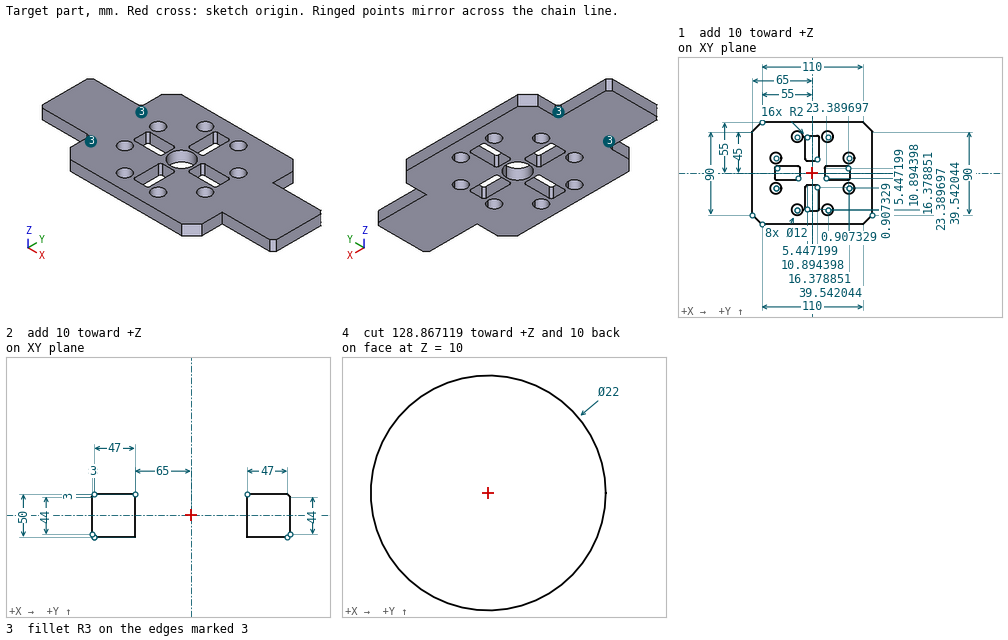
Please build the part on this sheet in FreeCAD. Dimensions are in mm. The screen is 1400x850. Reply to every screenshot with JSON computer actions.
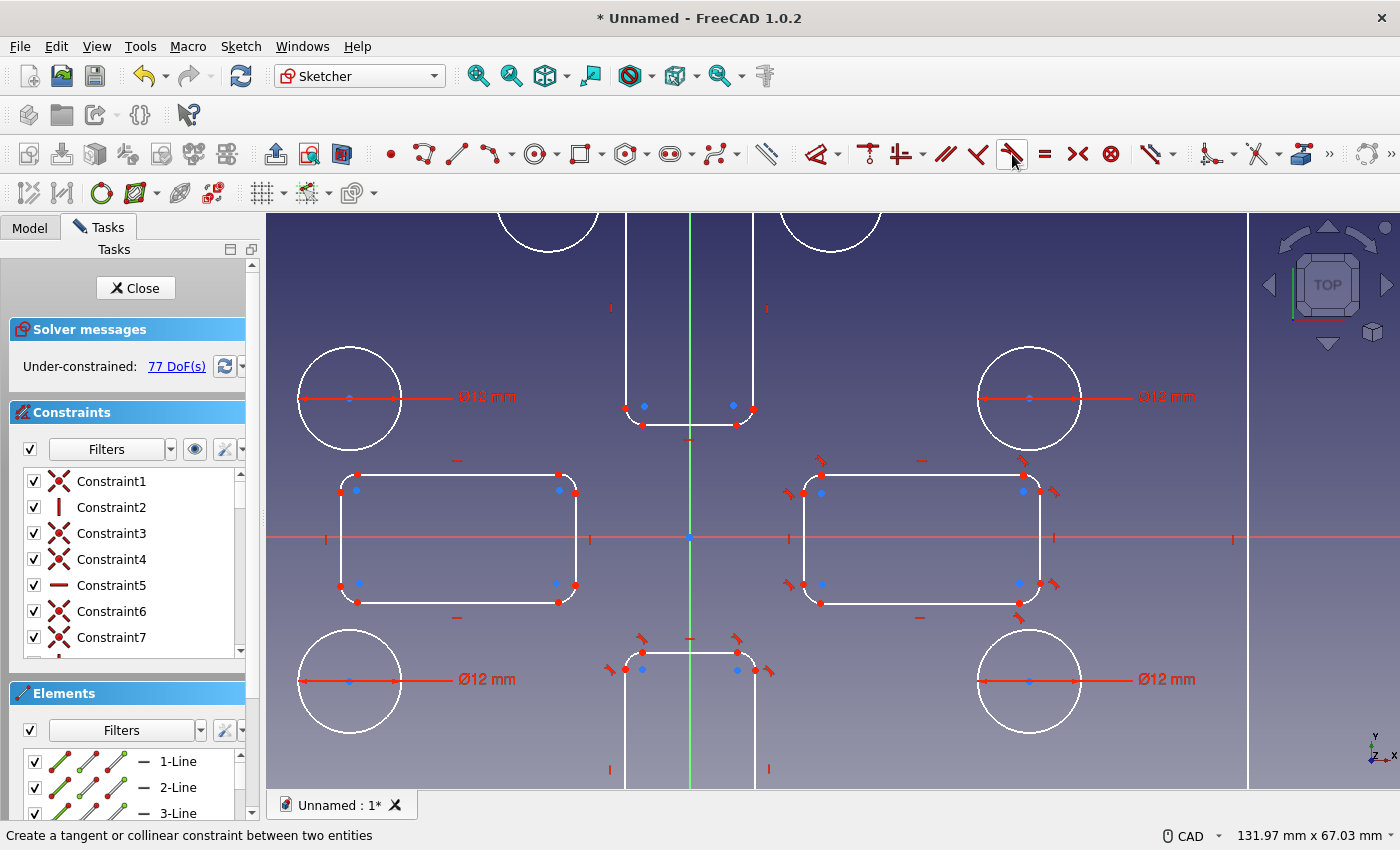
{"action": "left_click", "coordinate": [960, 604]}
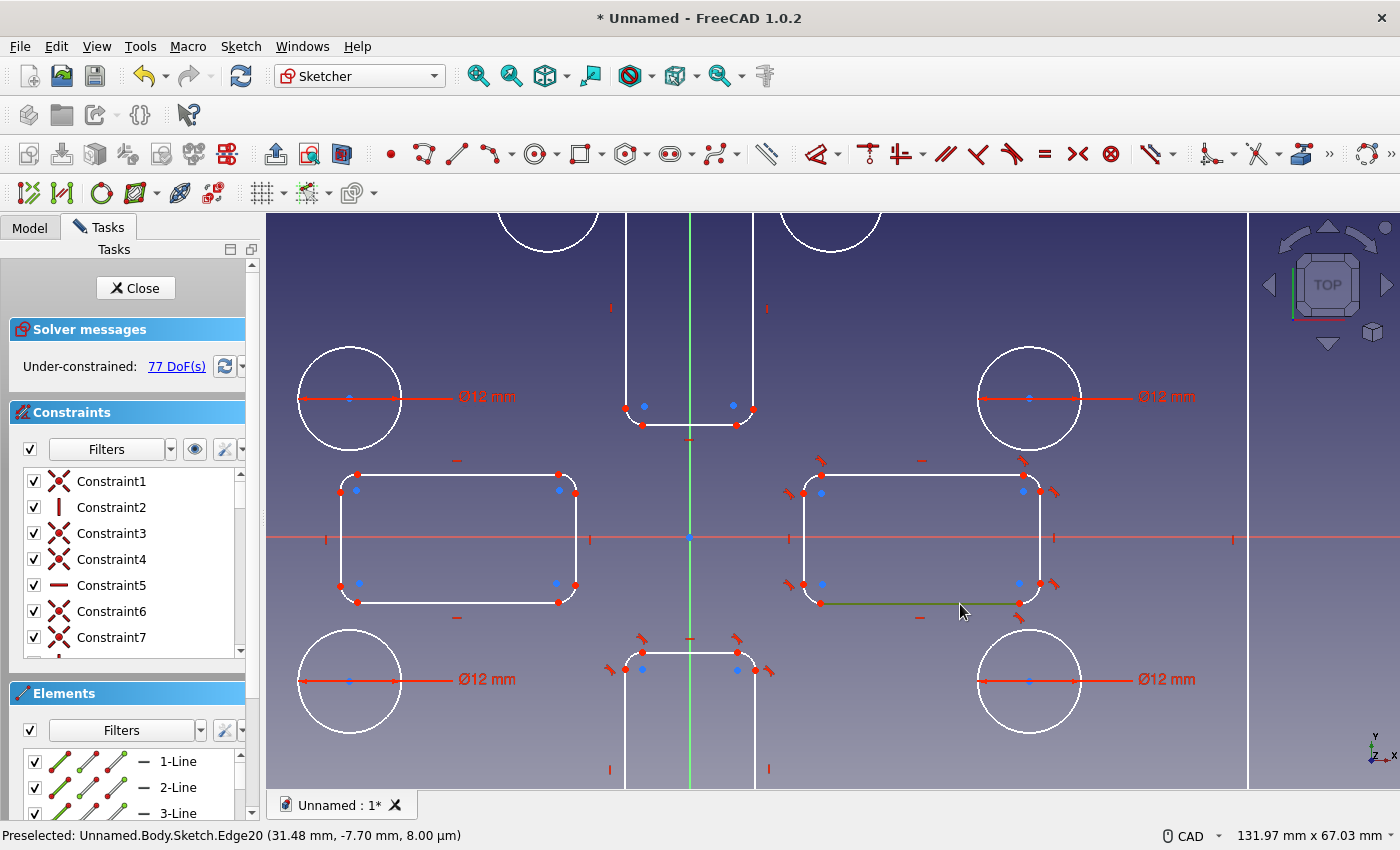
{"action": "left_click", "coordinate": [809, 597]}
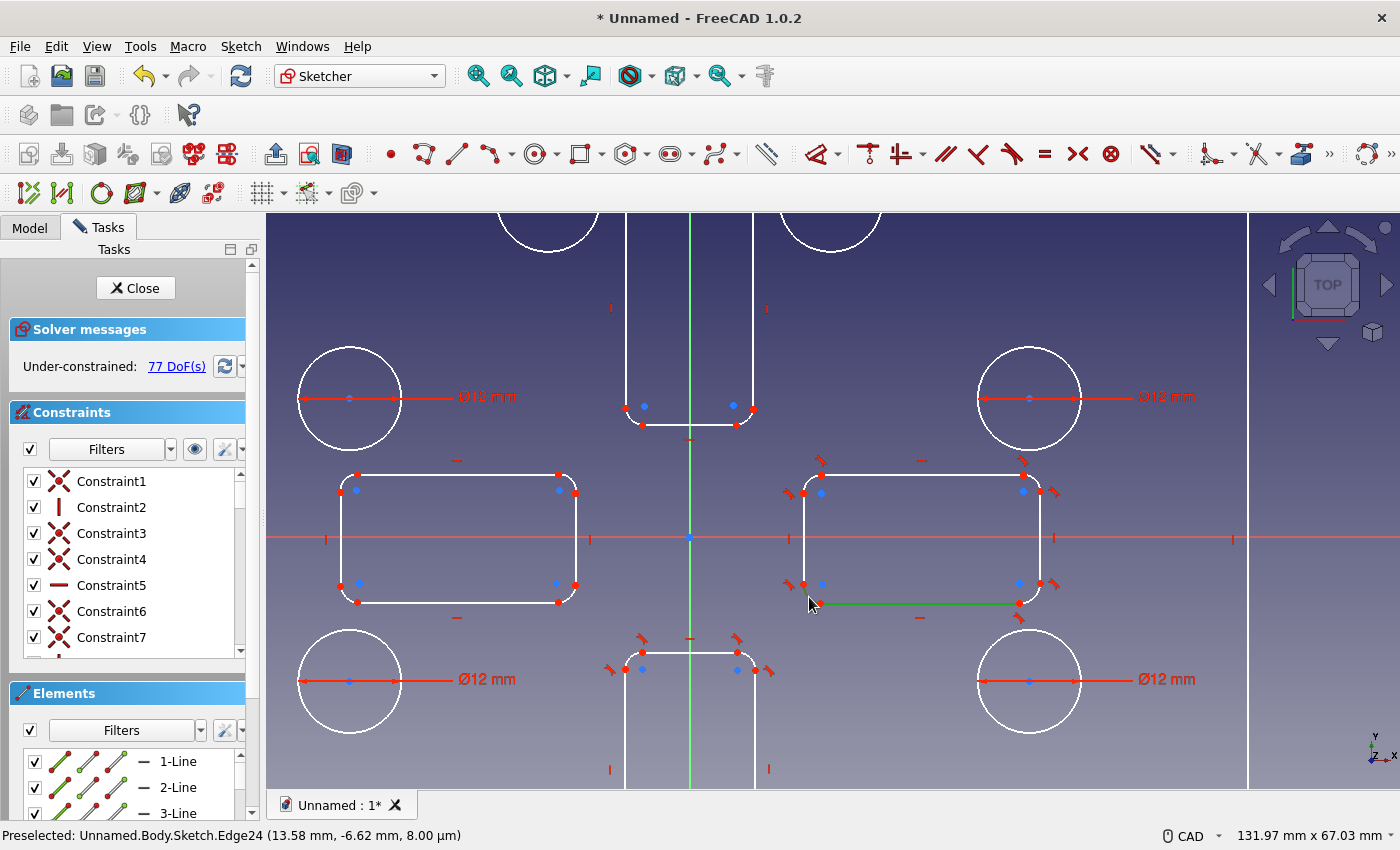
{"action": "left_click", "coordinate": [1012, 154]}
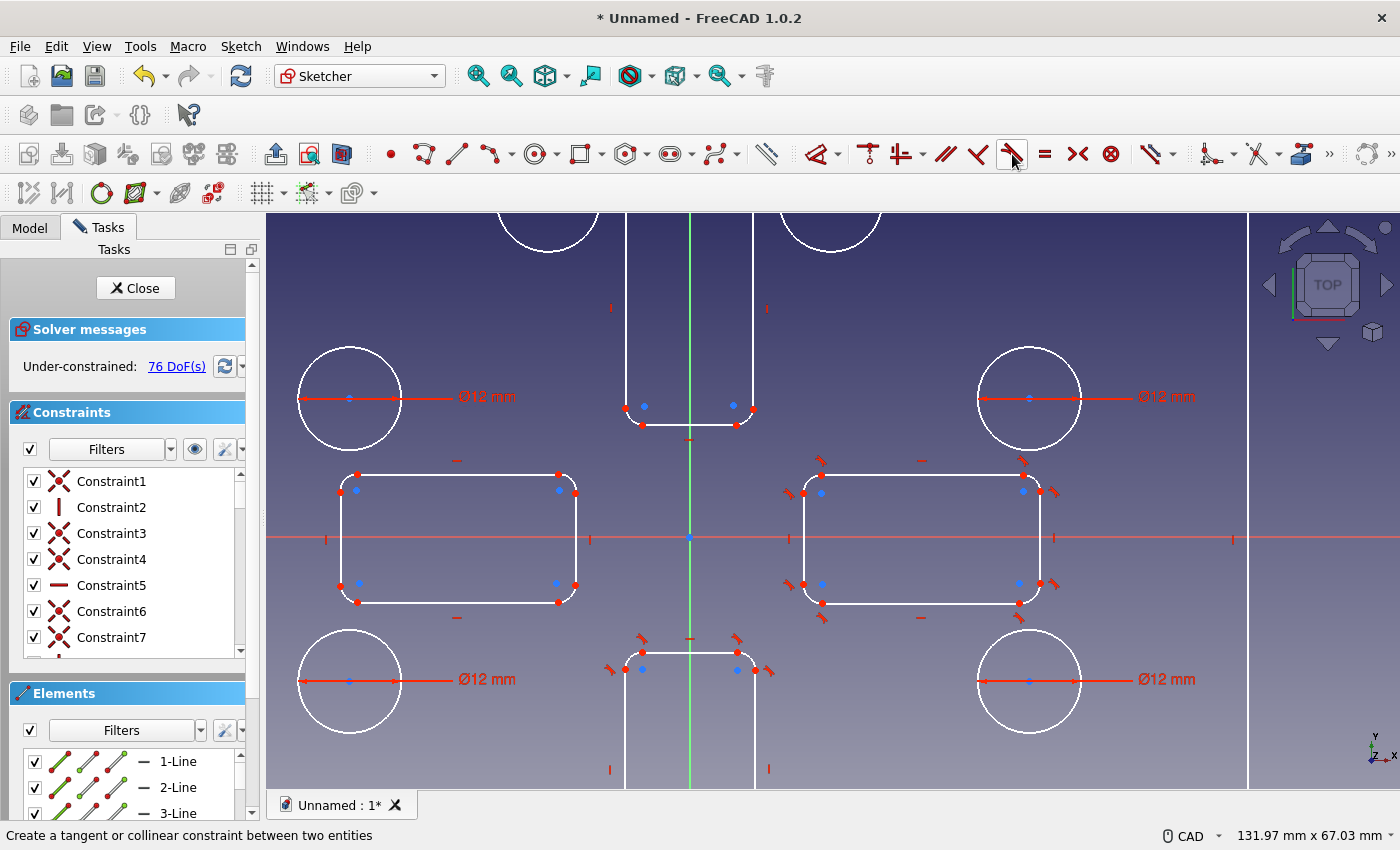
{"action": "left_click", "coordinate": [576, 521]}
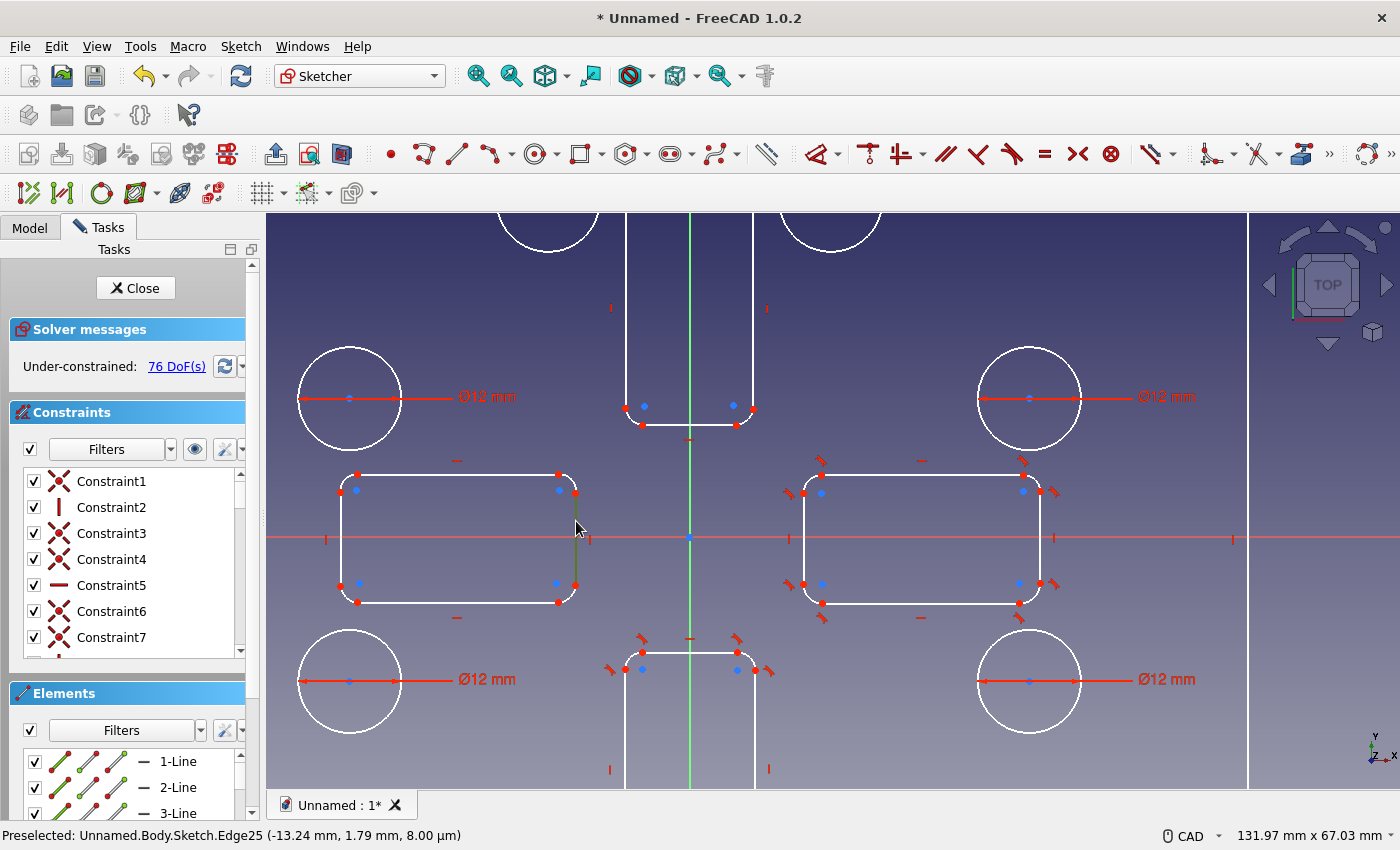
{"action": "left_click", "coordinate": [570, 597]}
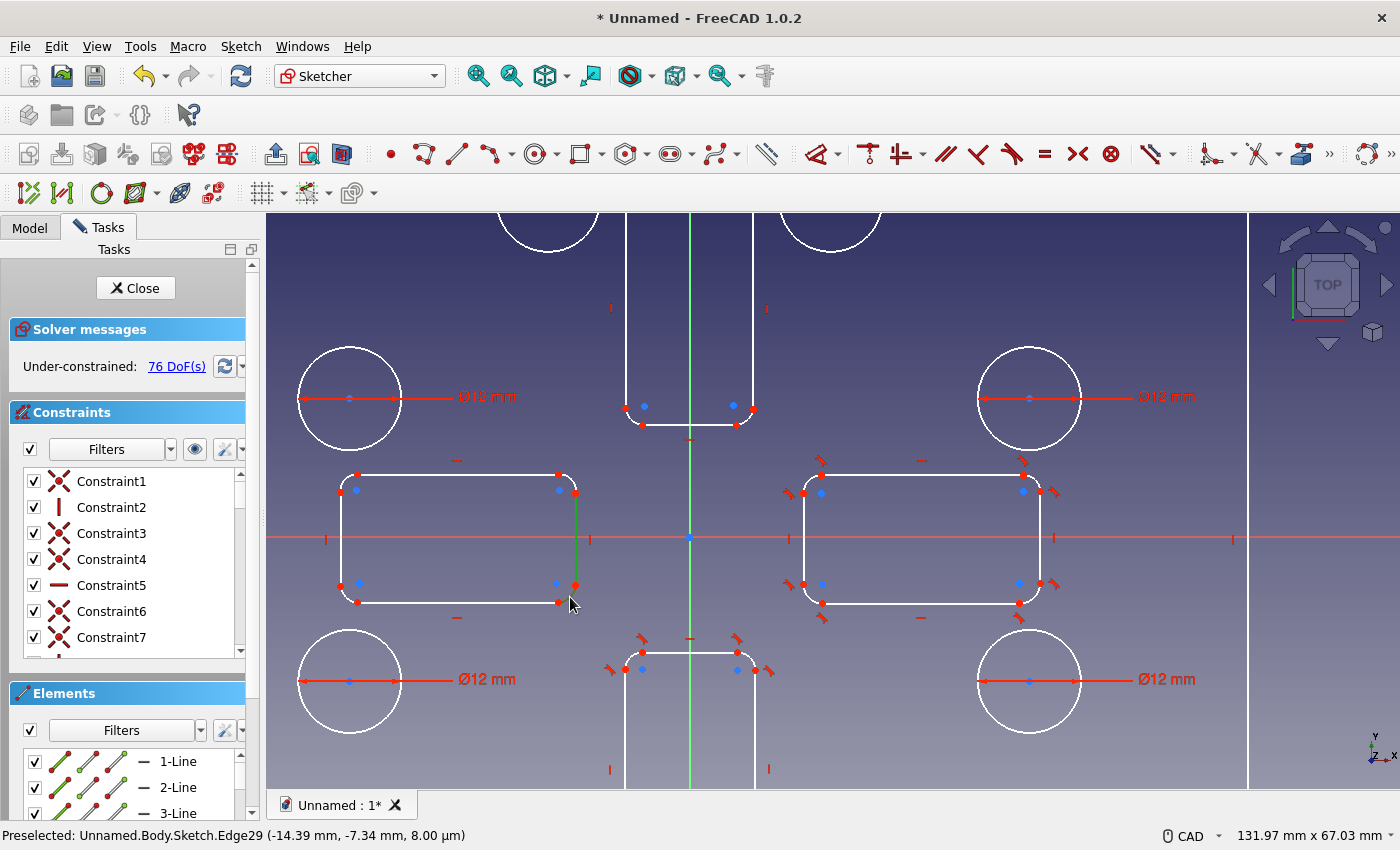
{"action": "left_click", "coordinate": [1012, 154]}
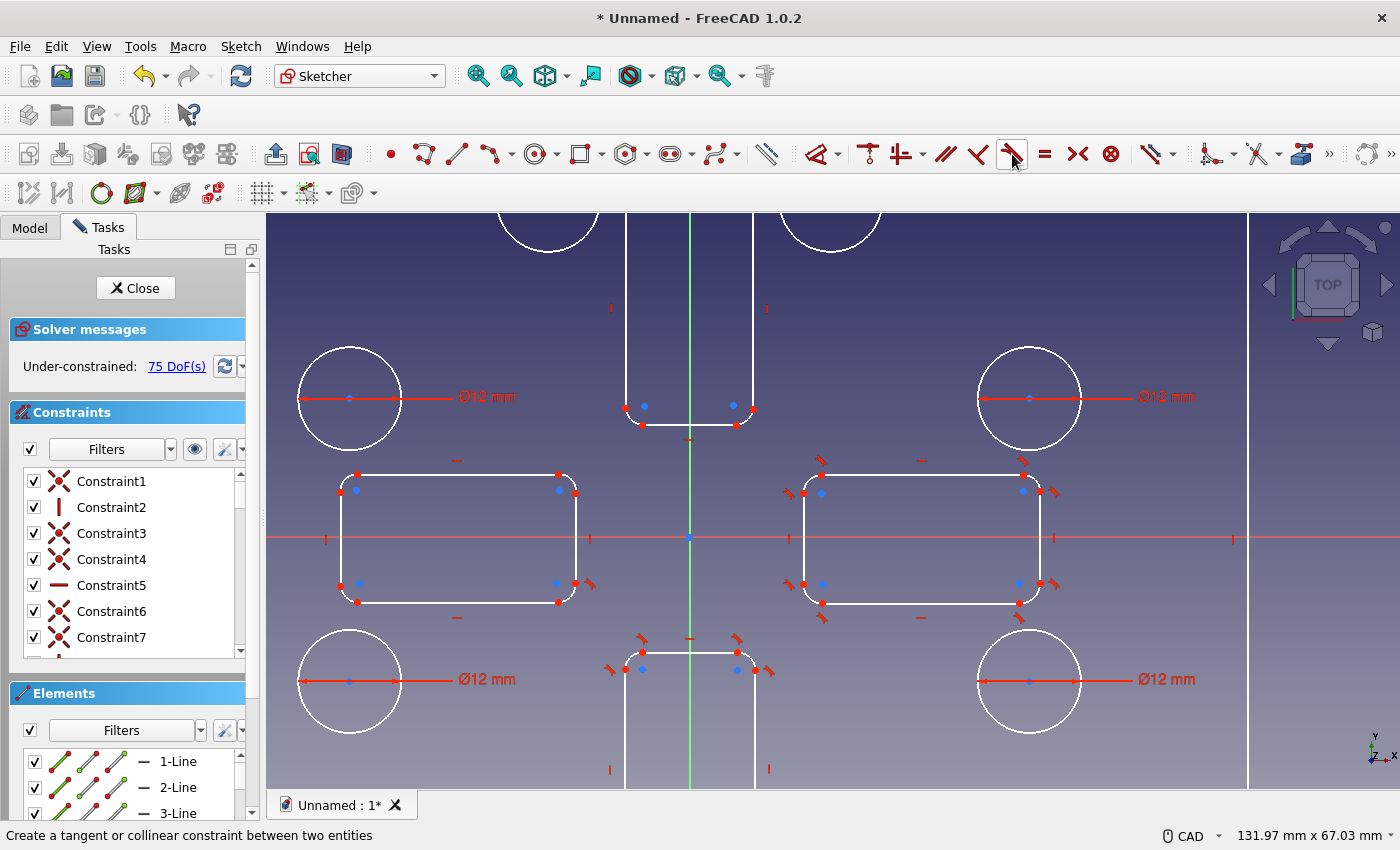
{"action": "left_click", "coordinate": [576, 520]}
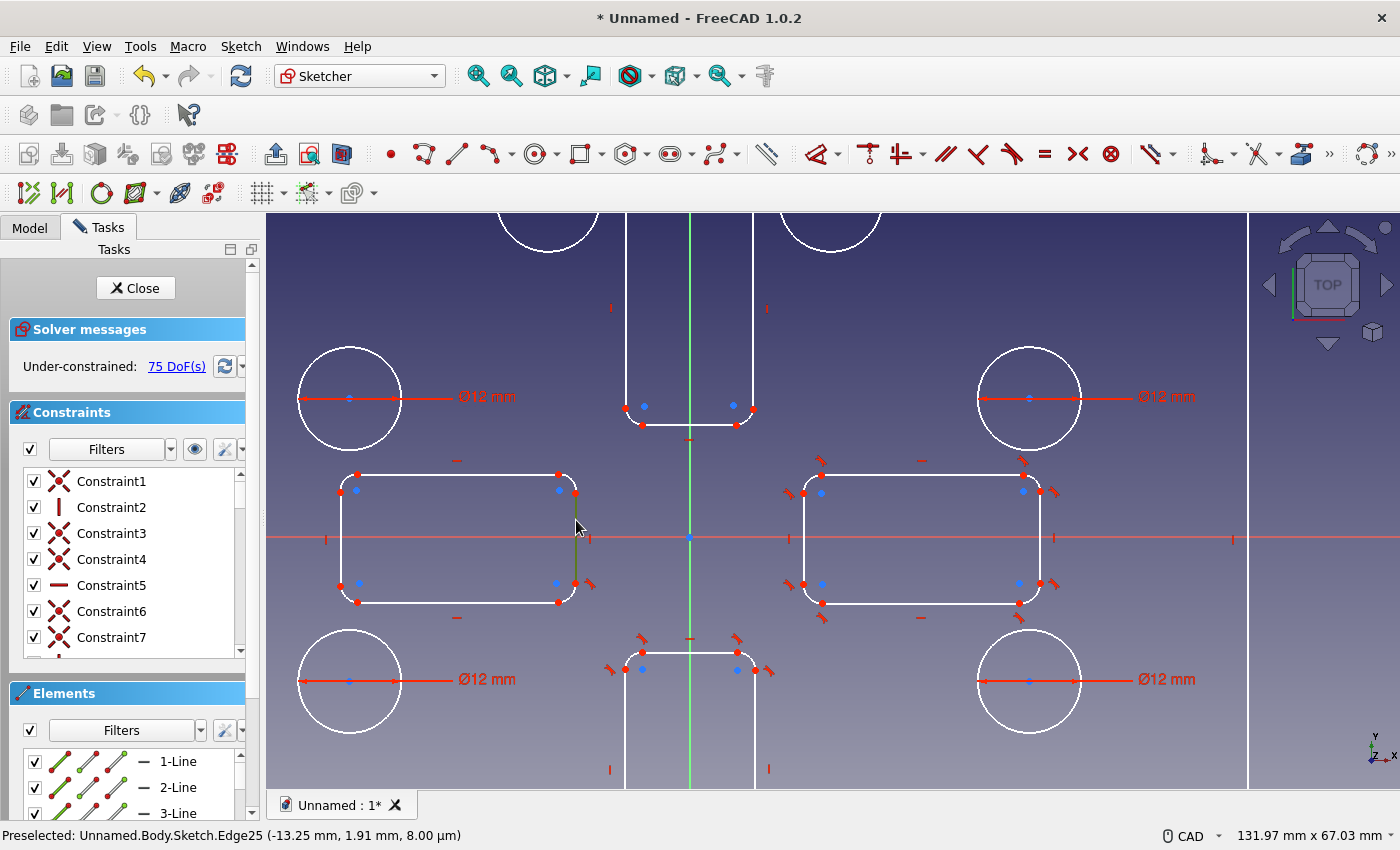
{"action": "left_click", "coordinate": [572, 480]}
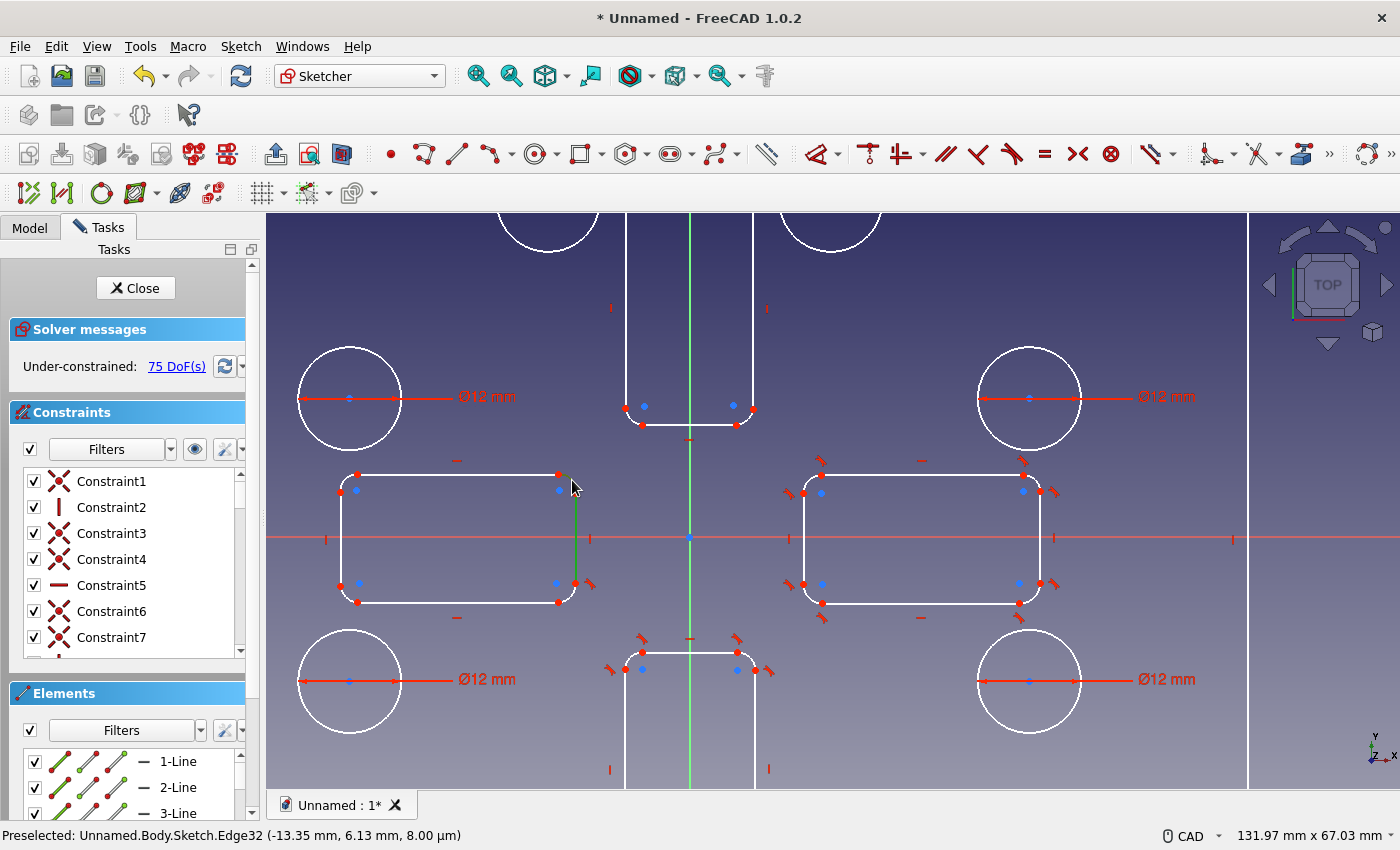
{"action": "left_click", "coordinate": [1012, 154]}